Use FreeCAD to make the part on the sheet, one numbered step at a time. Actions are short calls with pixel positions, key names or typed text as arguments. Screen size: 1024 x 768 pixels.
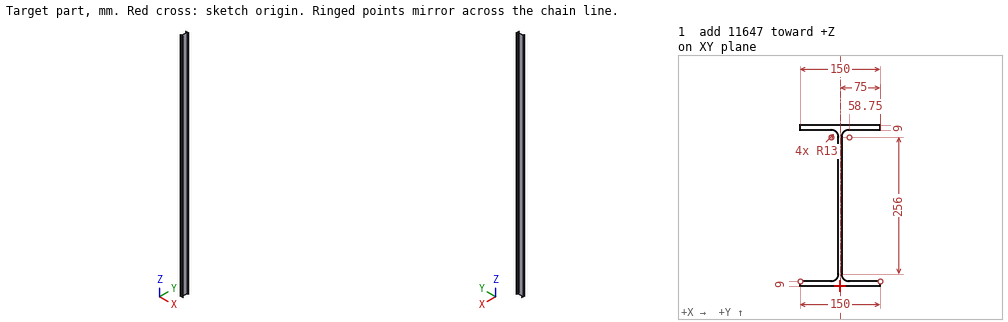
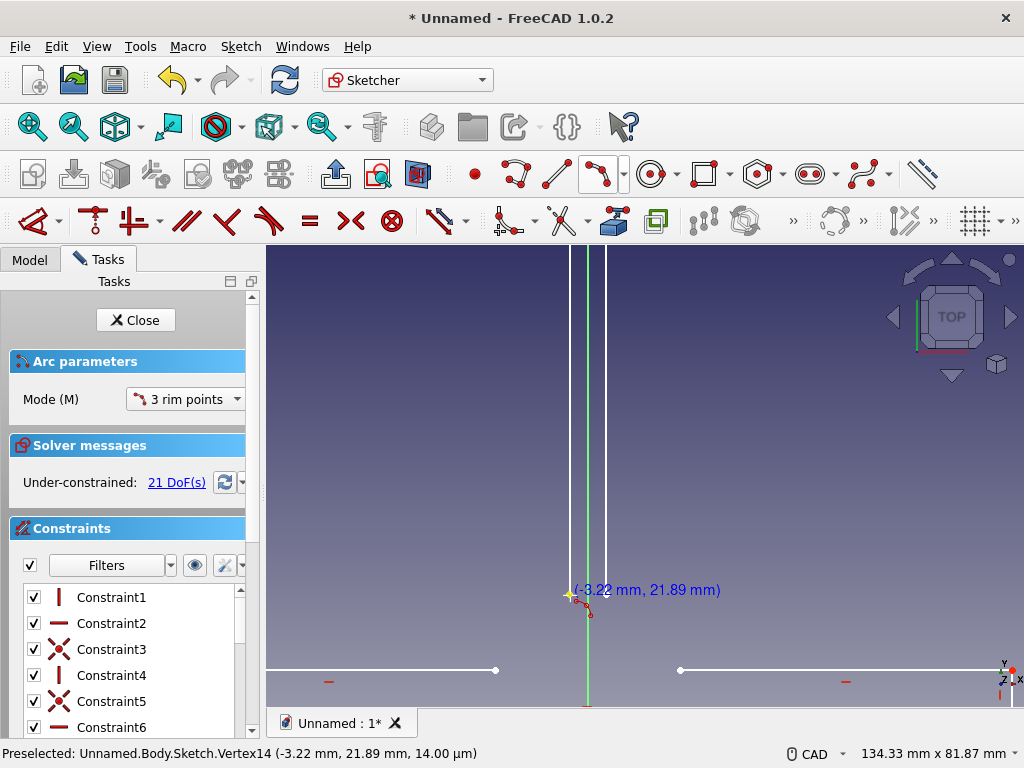
scroll(574, 596, down, 9)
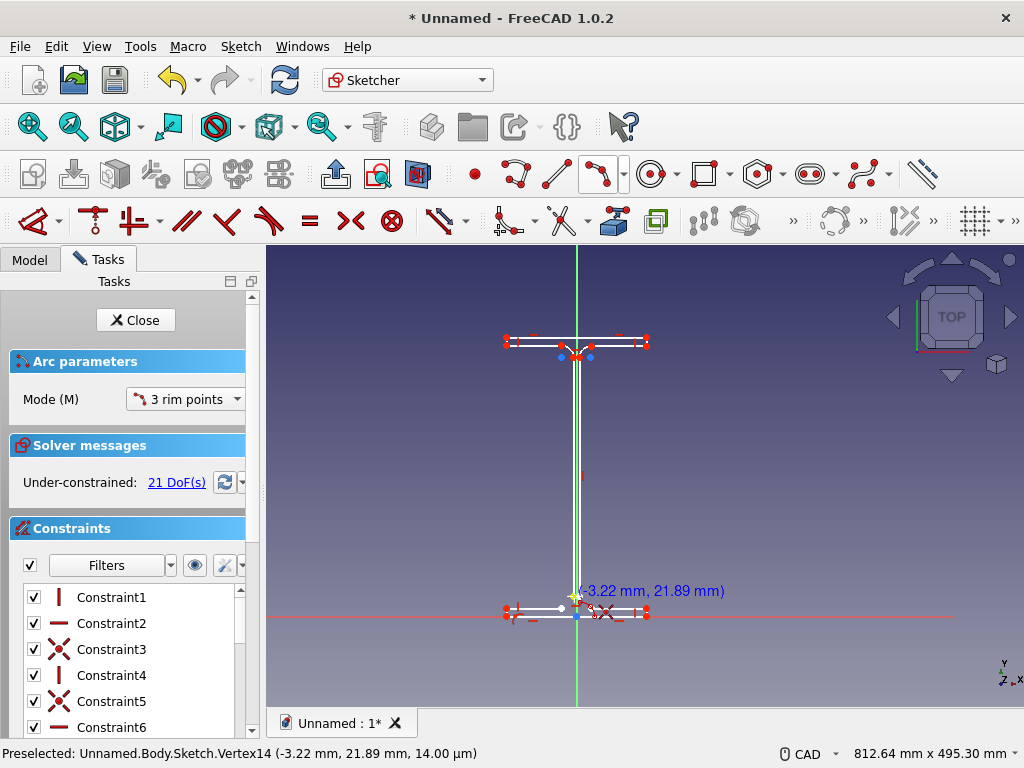
scroll(562, 608, up, 4)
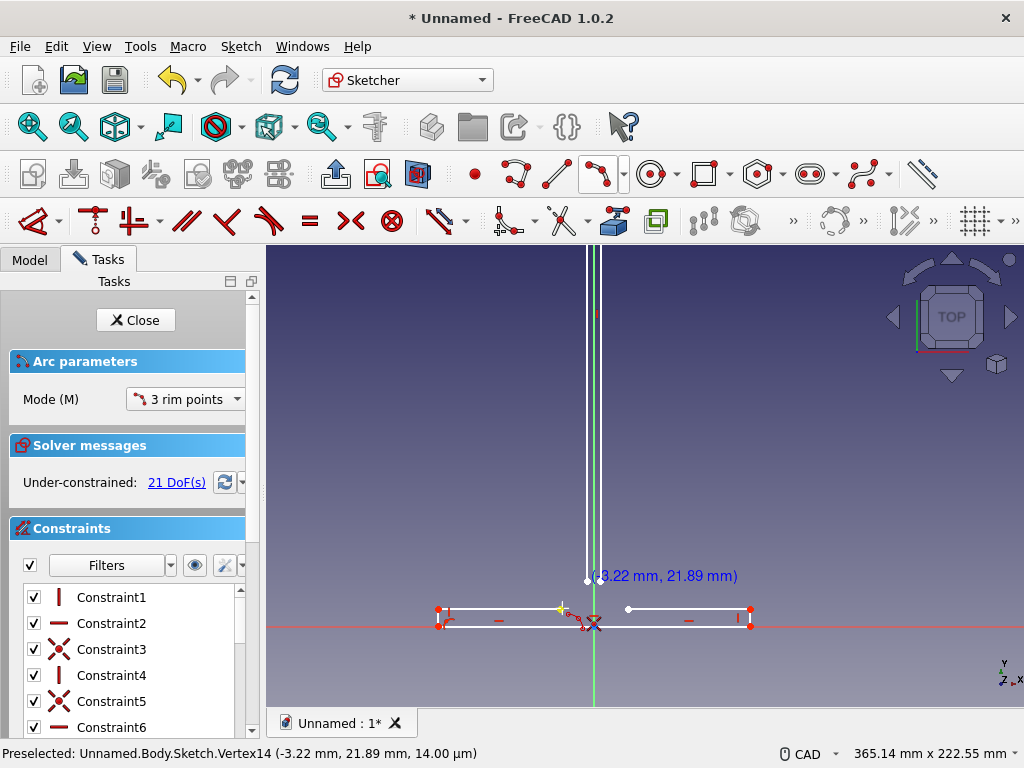
click(560, 609)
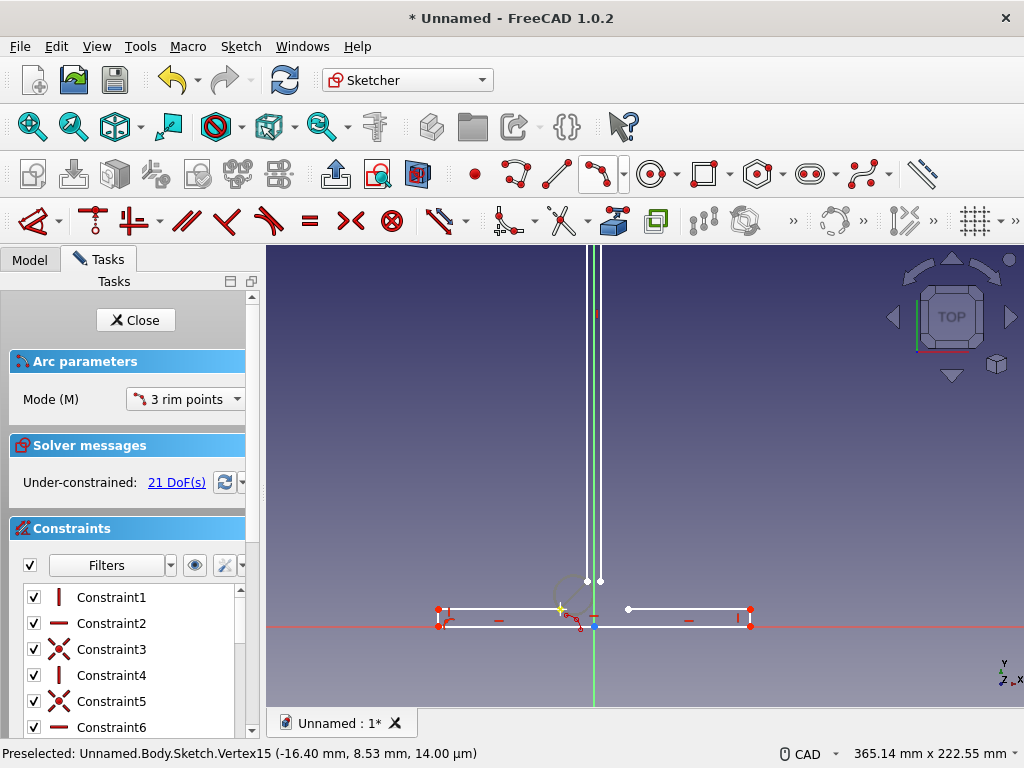
scroll(580, 600, up, 4)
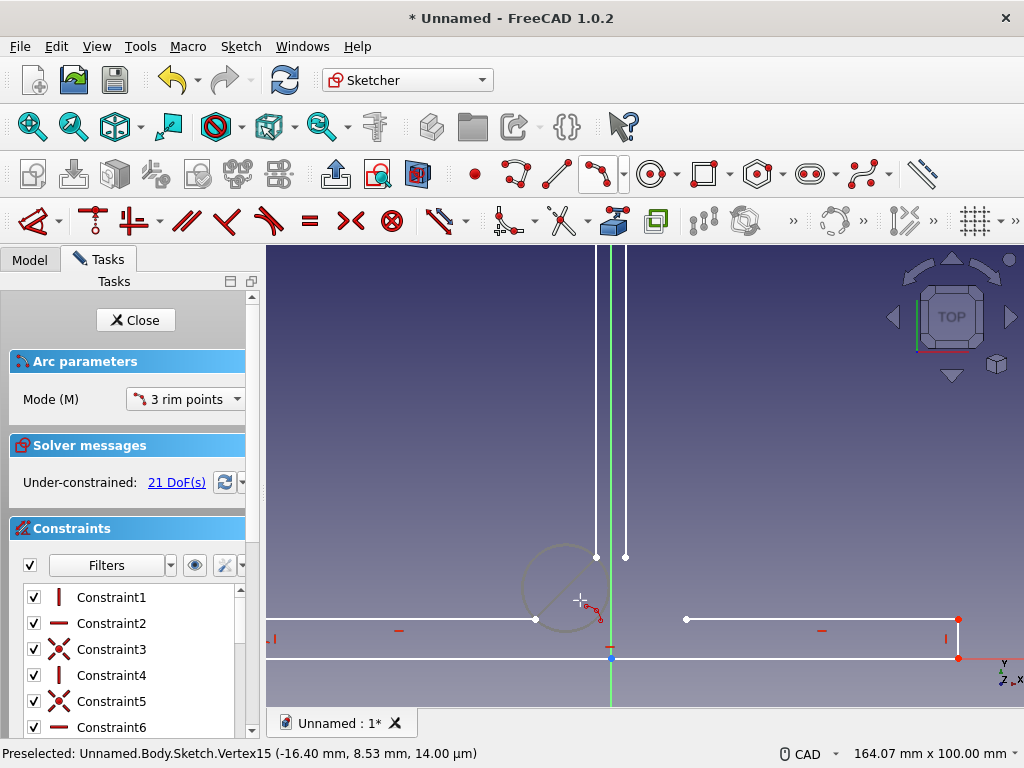
click(578, 599)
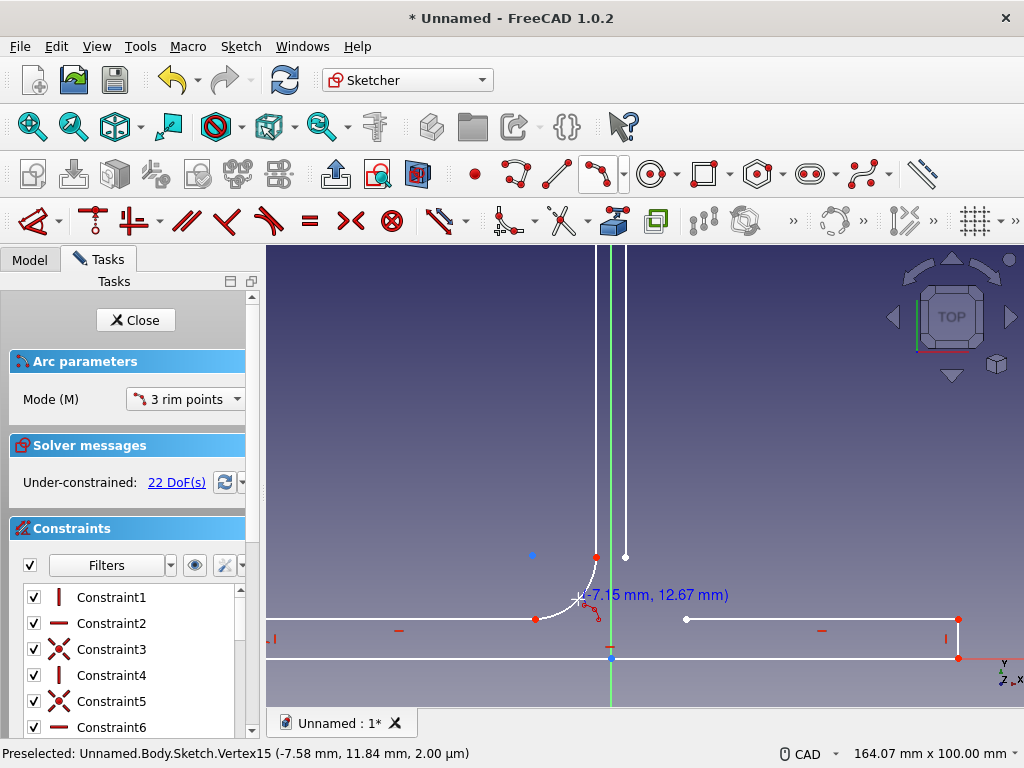
click(687, 619)
click(626, 558)
click(644, 599)
key(Escape)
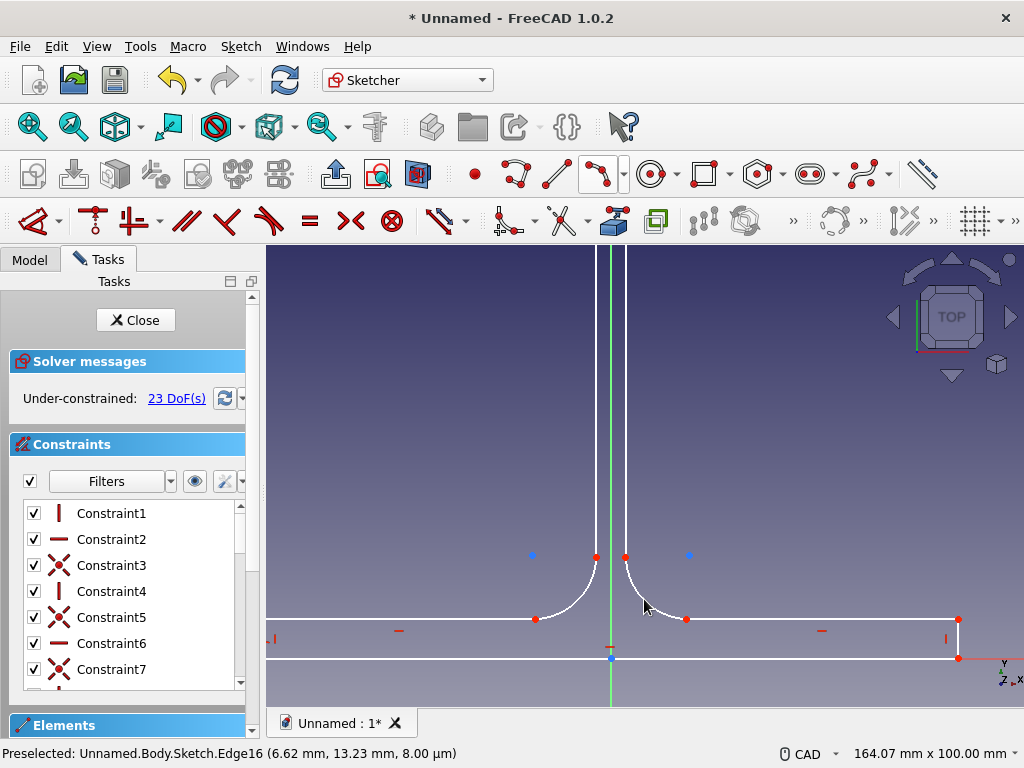
click(626, 321)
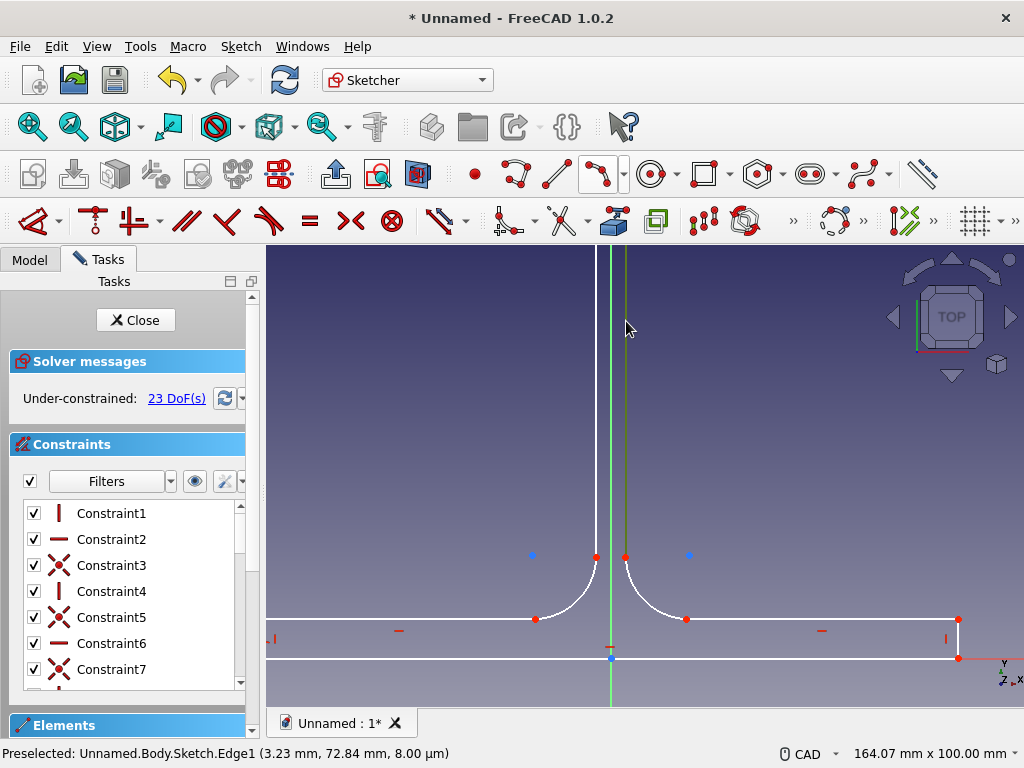
scroll(568, 605, down, 8)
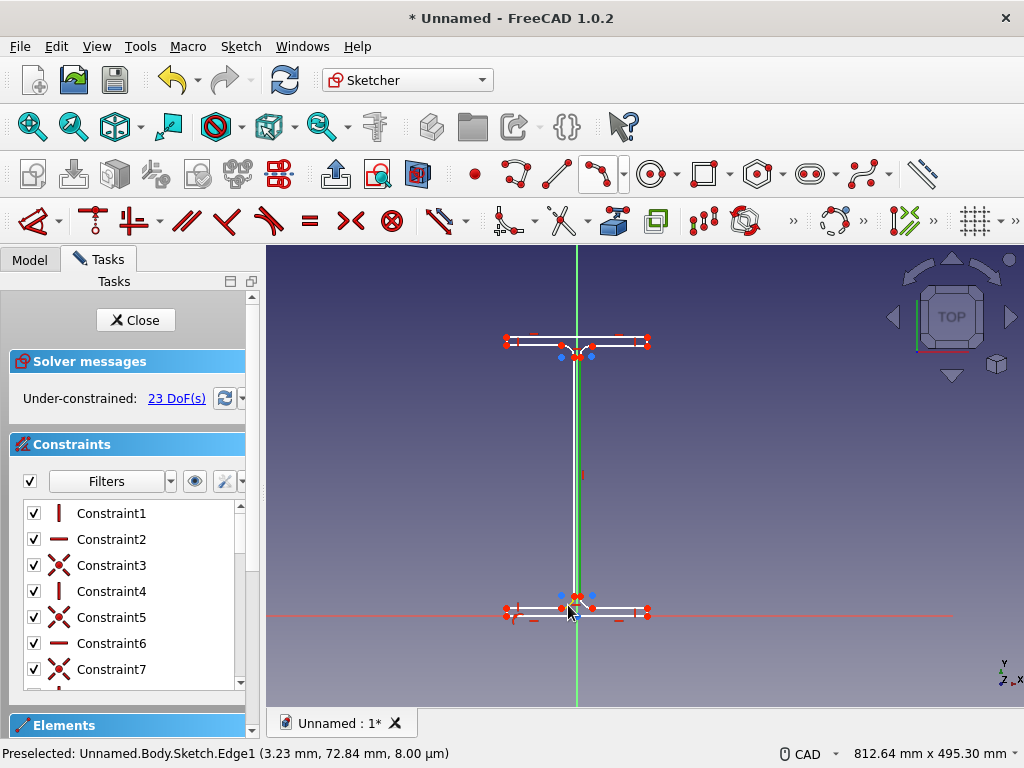
scroll(587, 347, up, 5)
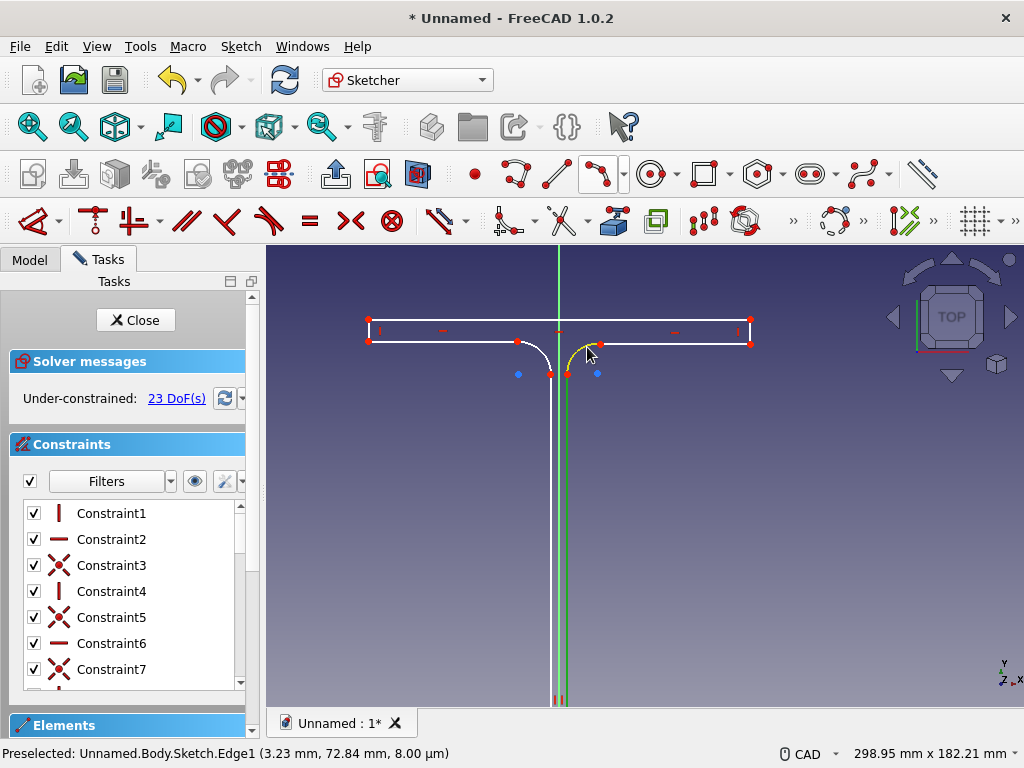
click(586, 346)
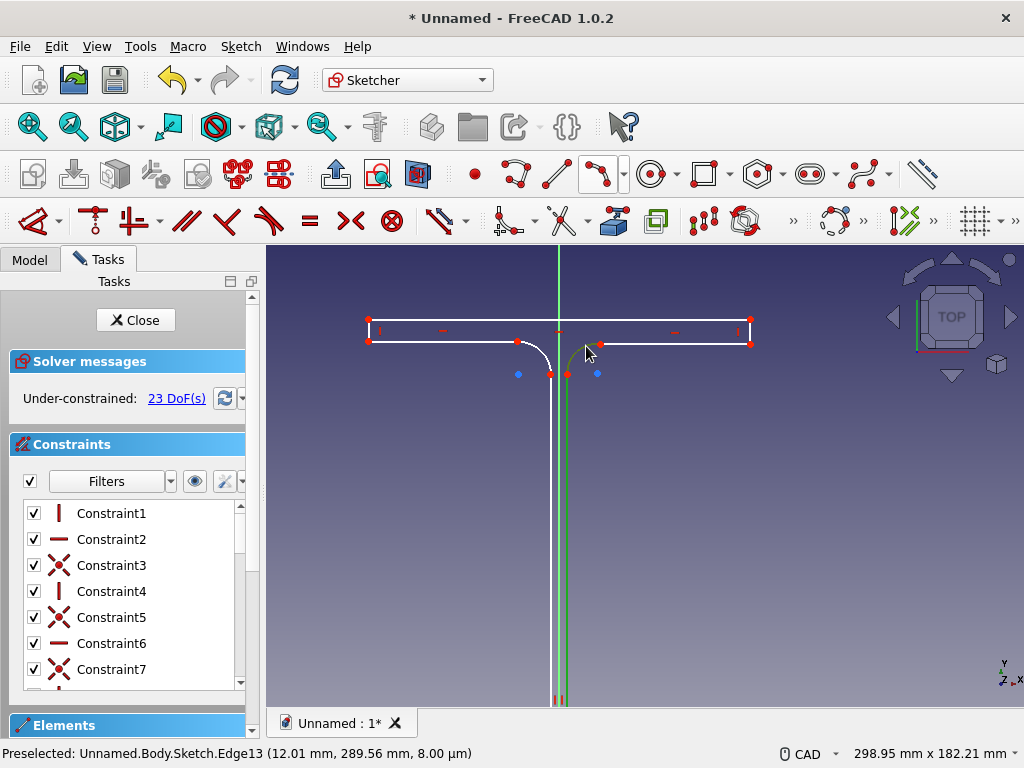
key(t)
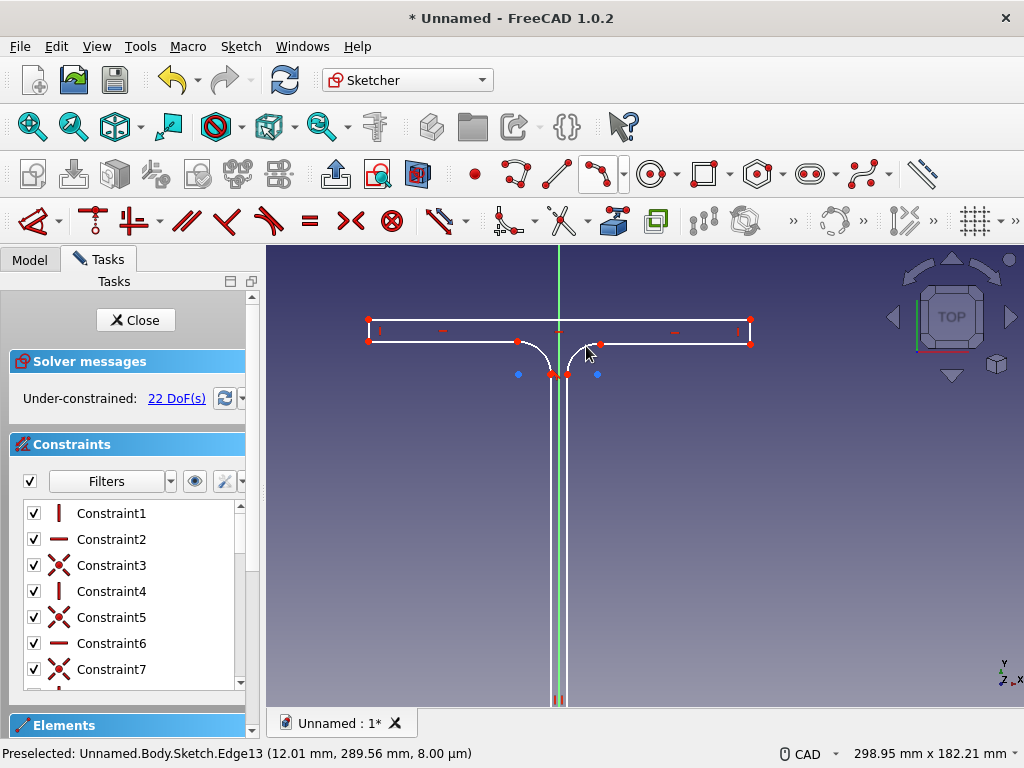
scroll(567, 569, up, 3)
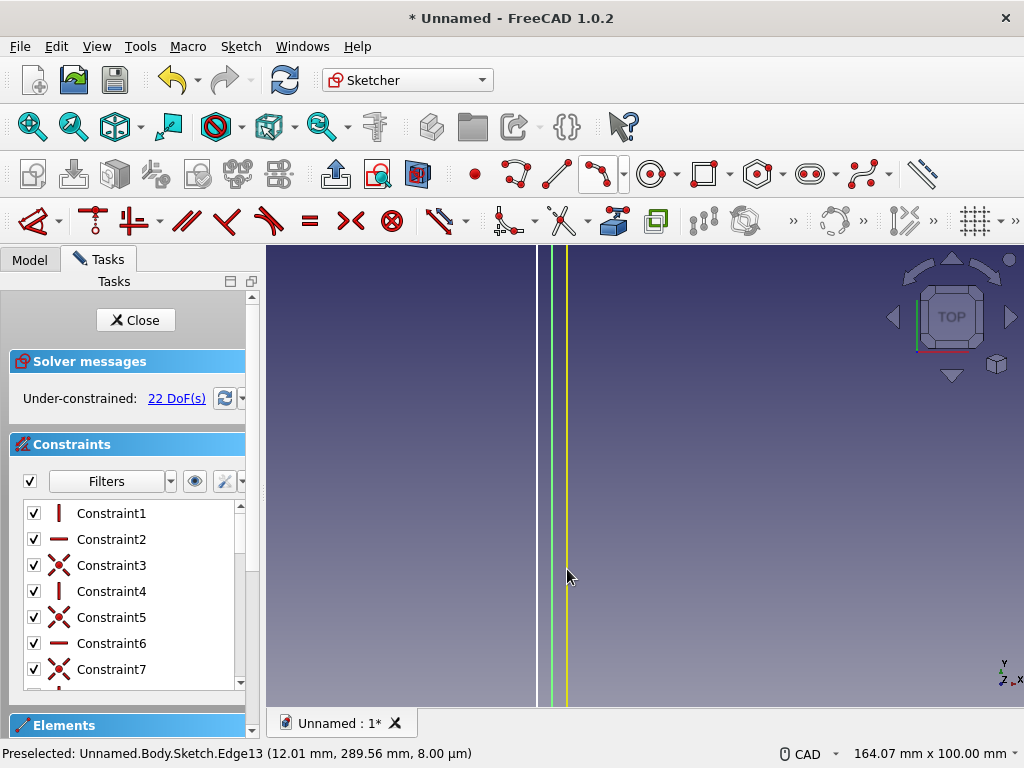
click(567, 569)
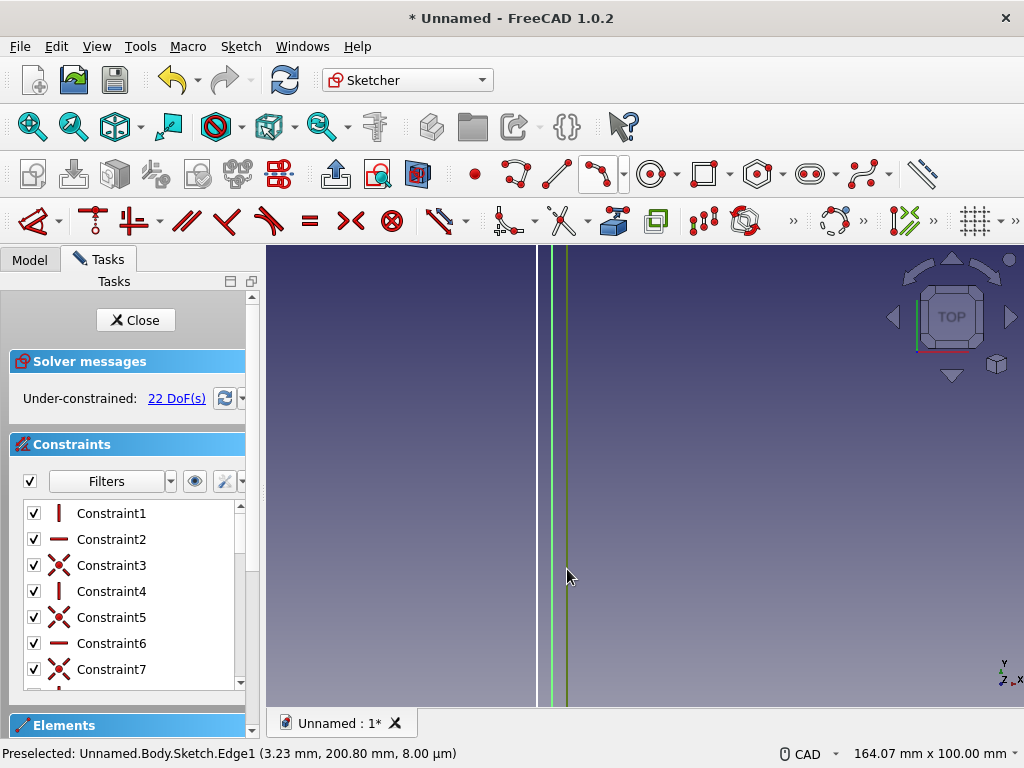
scroll(583, 393, down, 8)